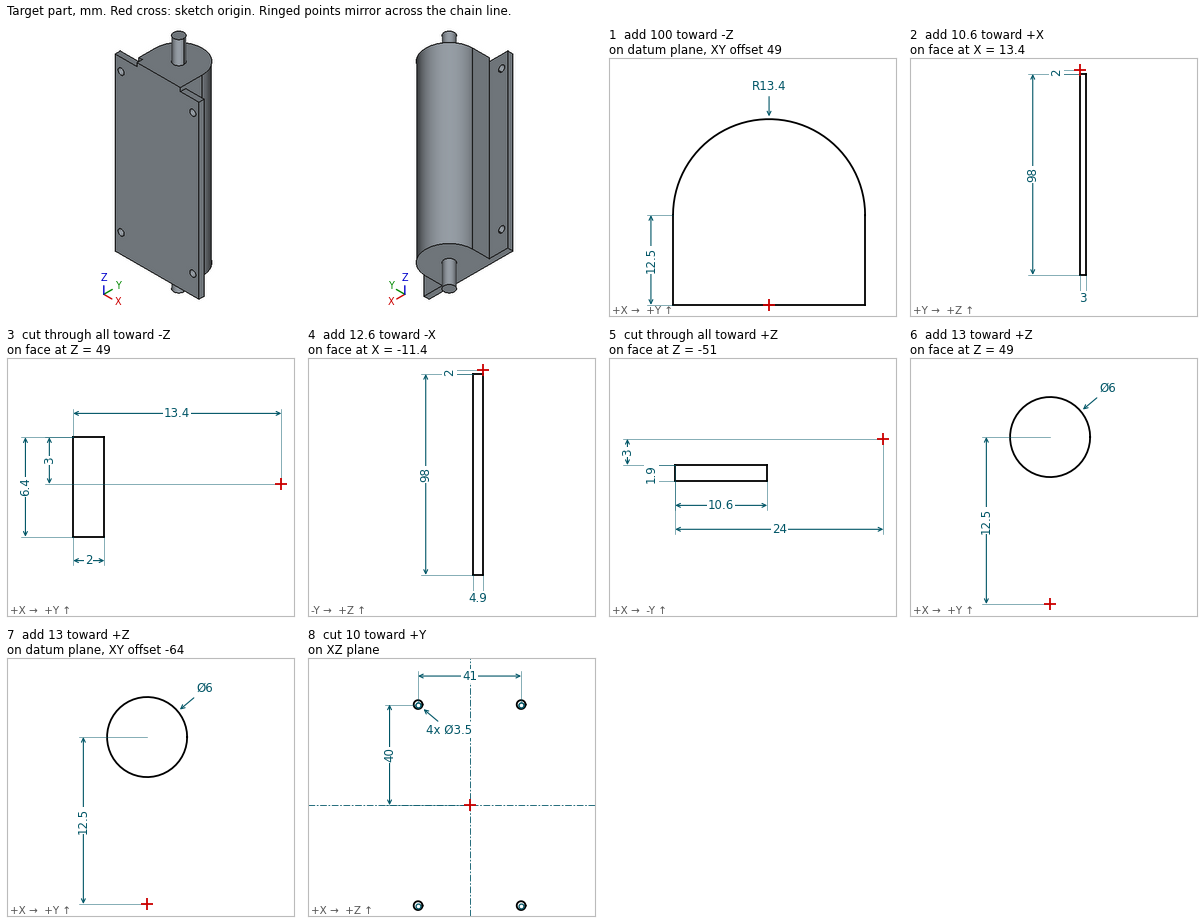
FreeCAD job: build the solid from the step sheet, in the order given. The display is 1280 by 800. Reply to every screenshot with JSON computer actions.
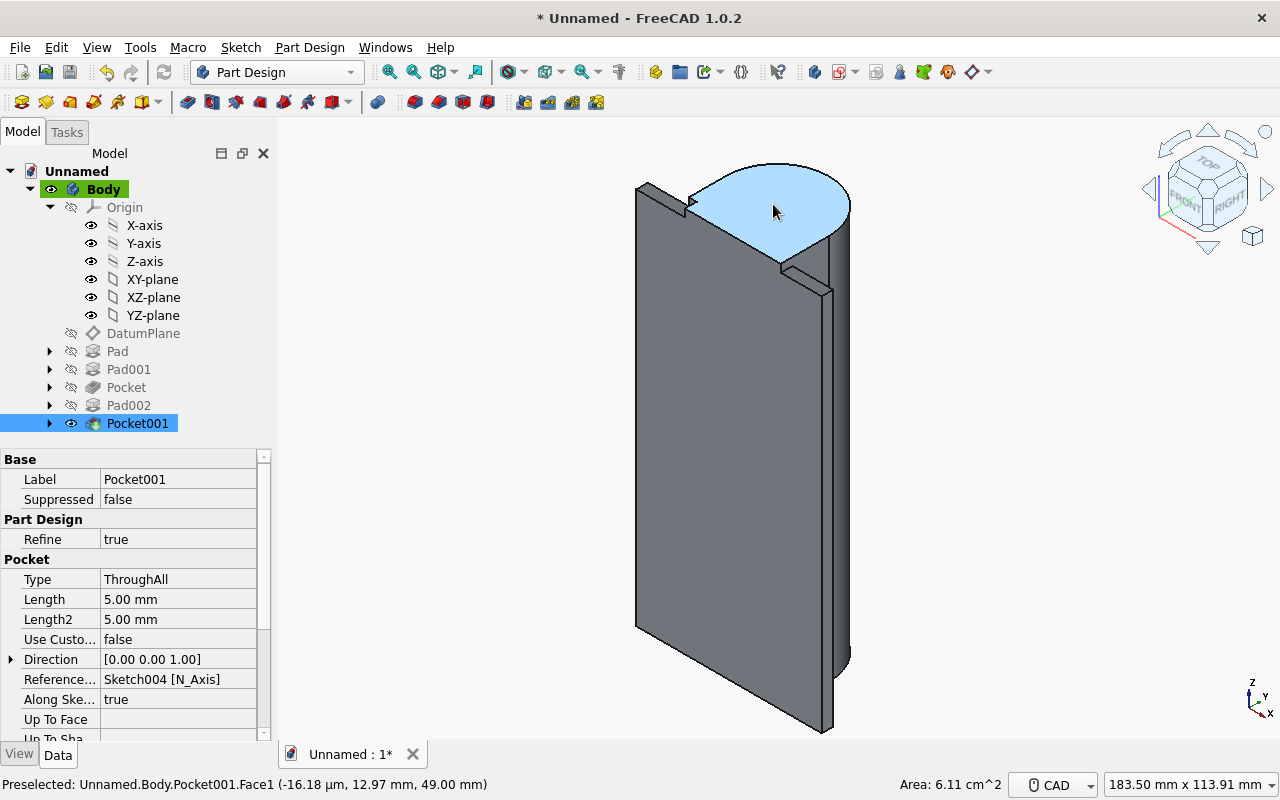
{"action": "left_click", "coordinate": [840, 72]}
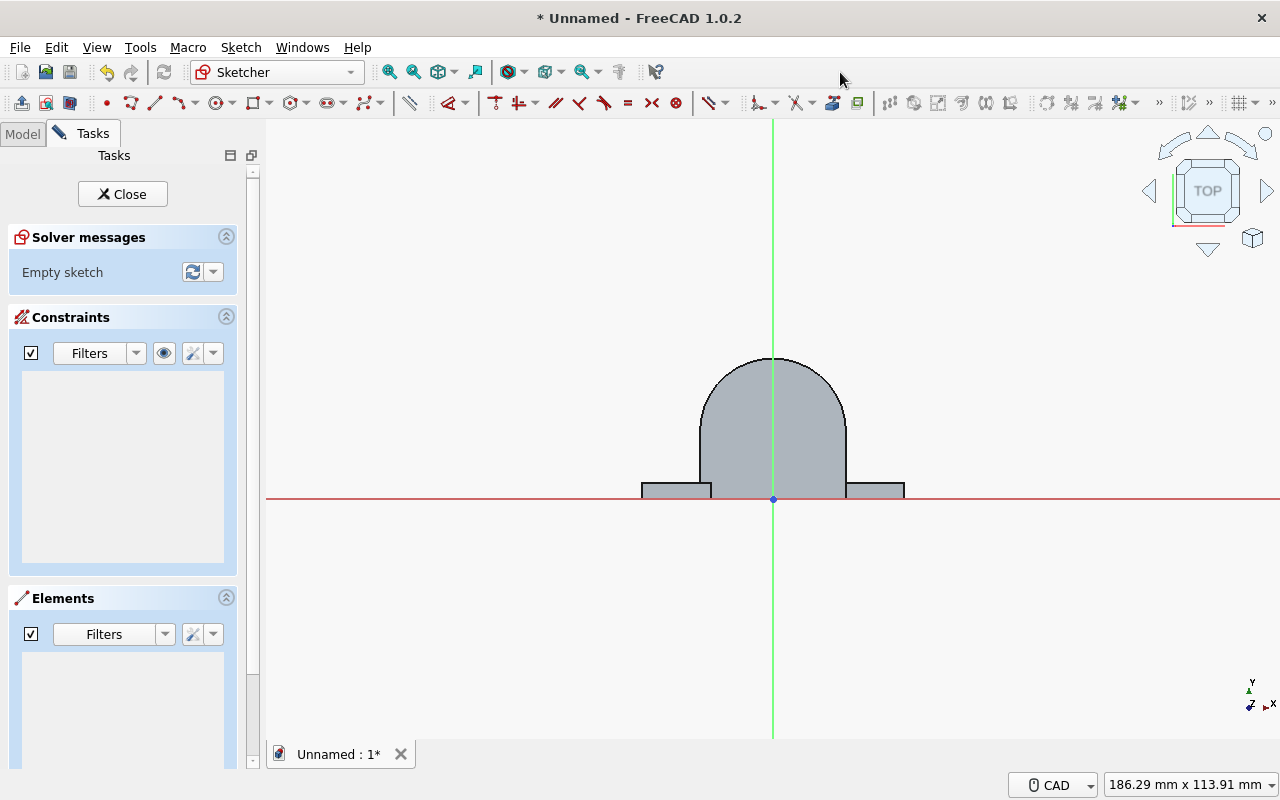
{"action": "scroll", "coordinate": [778, 432], "scroll_direction": "up", "scroll_amount": 13}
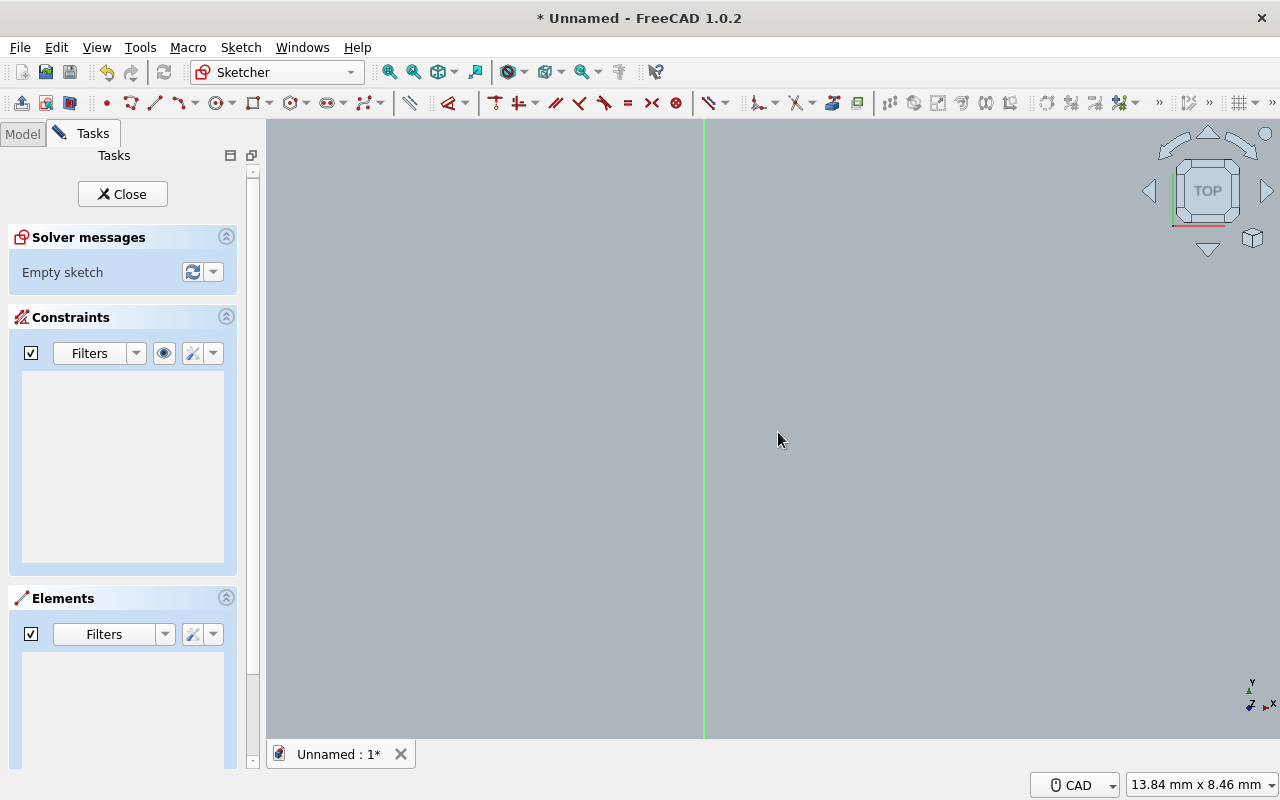
{"action": "left_click", "coordinate": [216, 104]}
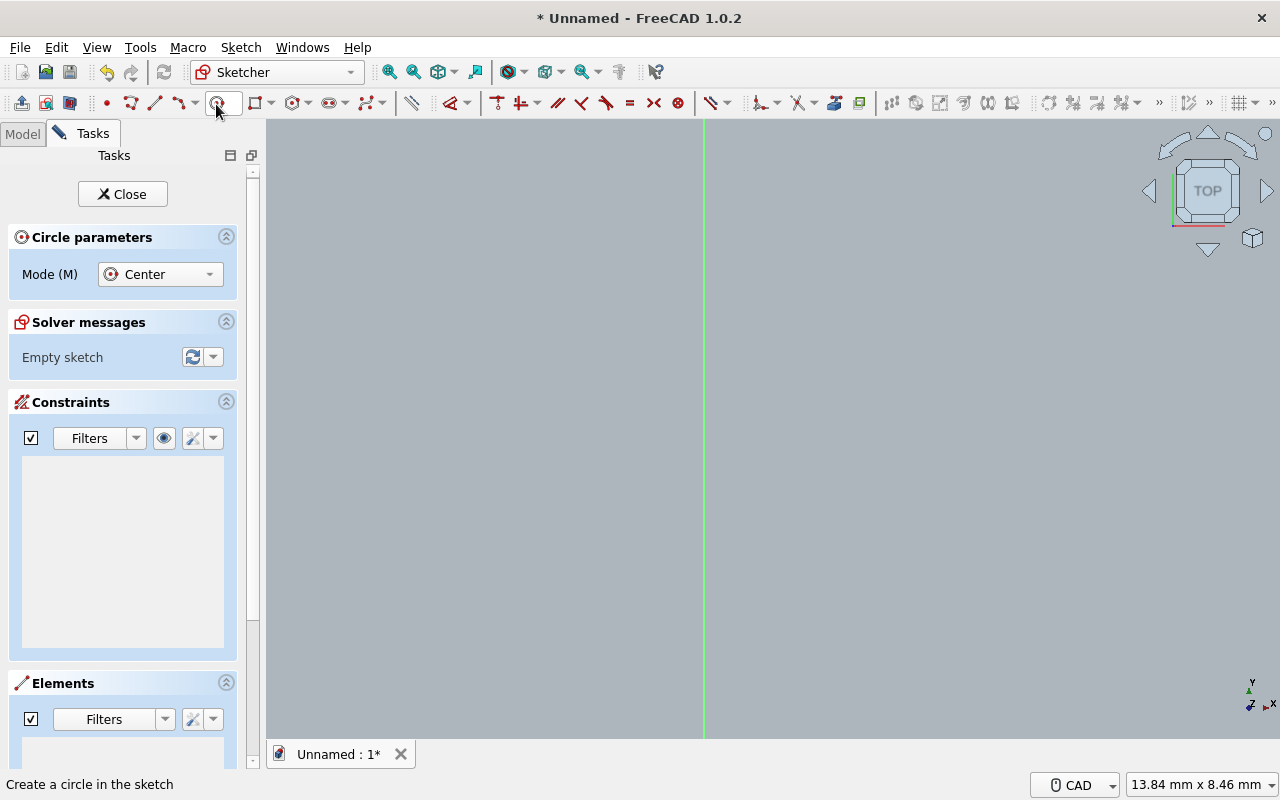
{"action": "left_click", "coordinate": [704, 418]}
{"action": "left_click", "coordinate": [860, 263]}
{"action": "key", "text": "Escape"}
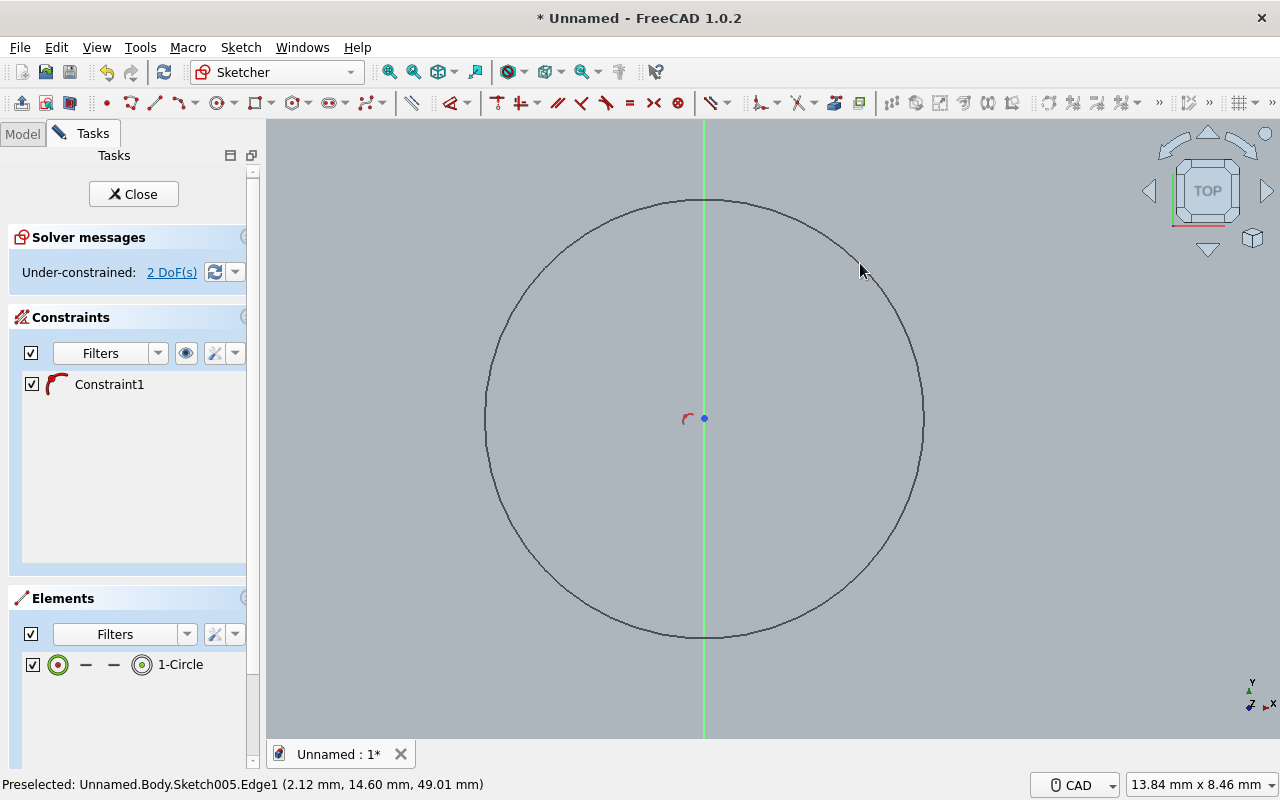
{"action": "left_click", "coordinate": [450, 104]}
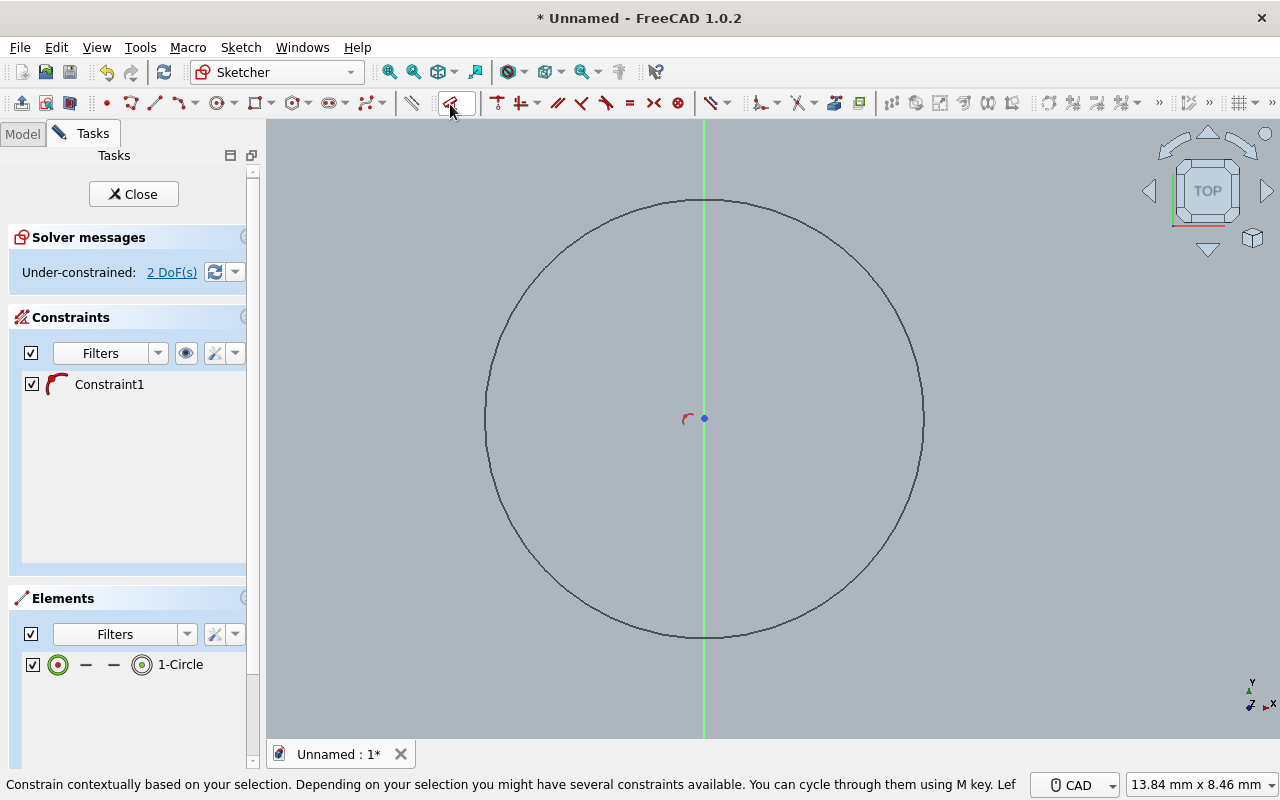
{"action": "left_click", "coordinate": [859, 263]}
{"action": "left_click", "coordinate": [882, 240]}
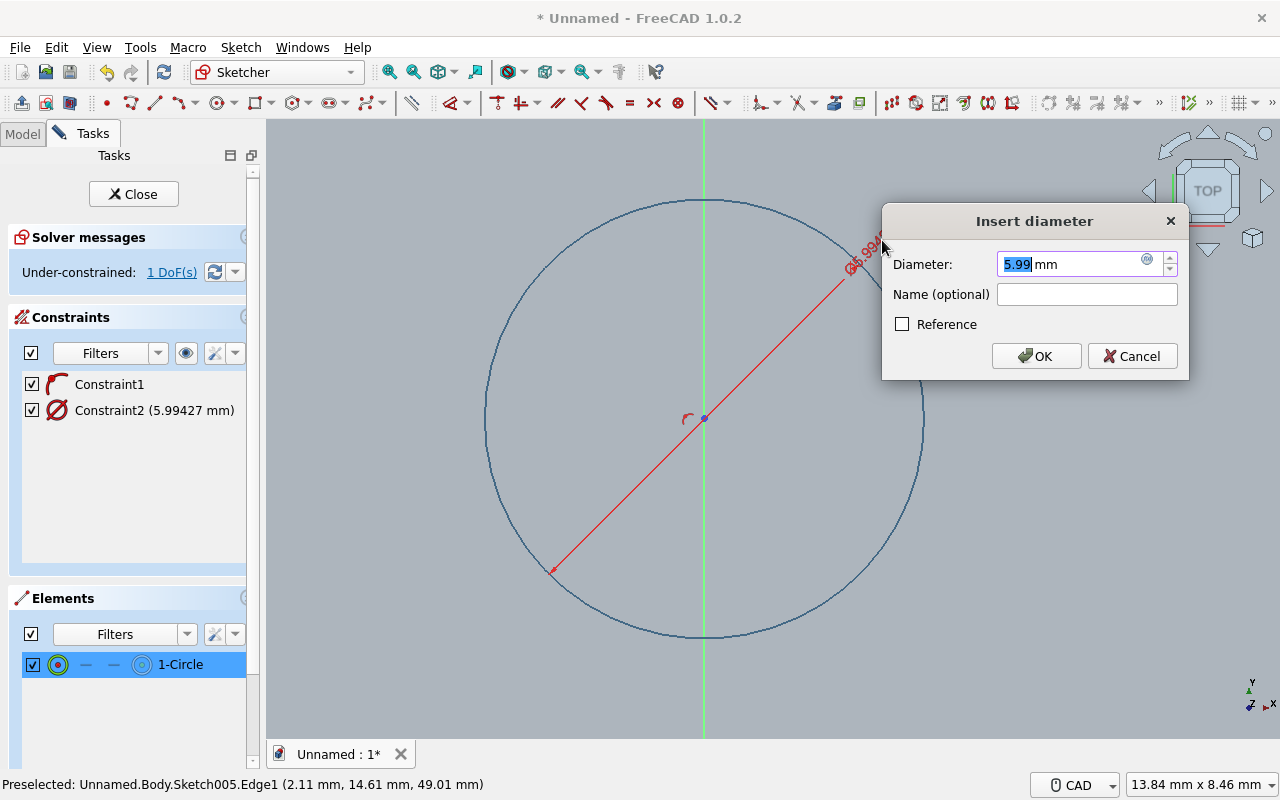
{"action": "type", "text": "6"}
{"action": "key", "text": "Return"}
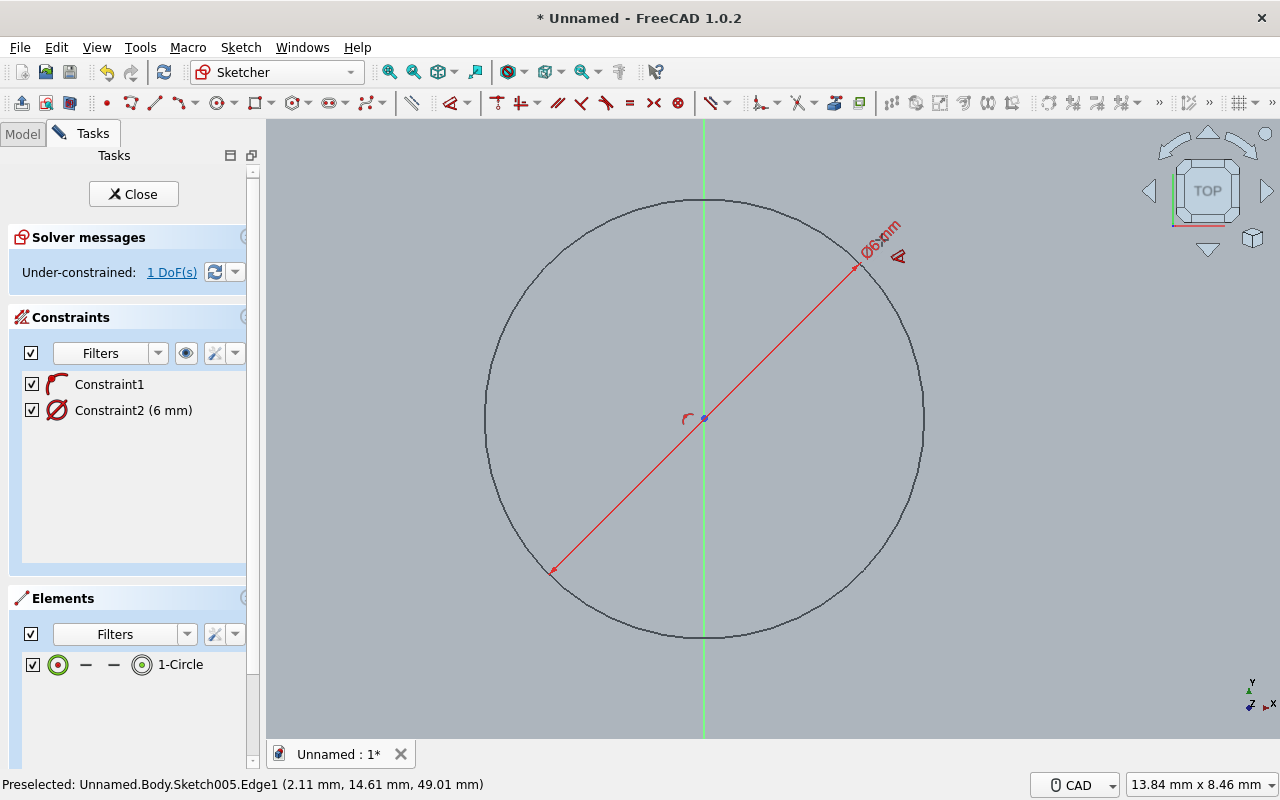
{"action": "left_click", "coordinate": [704, 419]}
{"action": "left_click", "coordinate": [738, 565]}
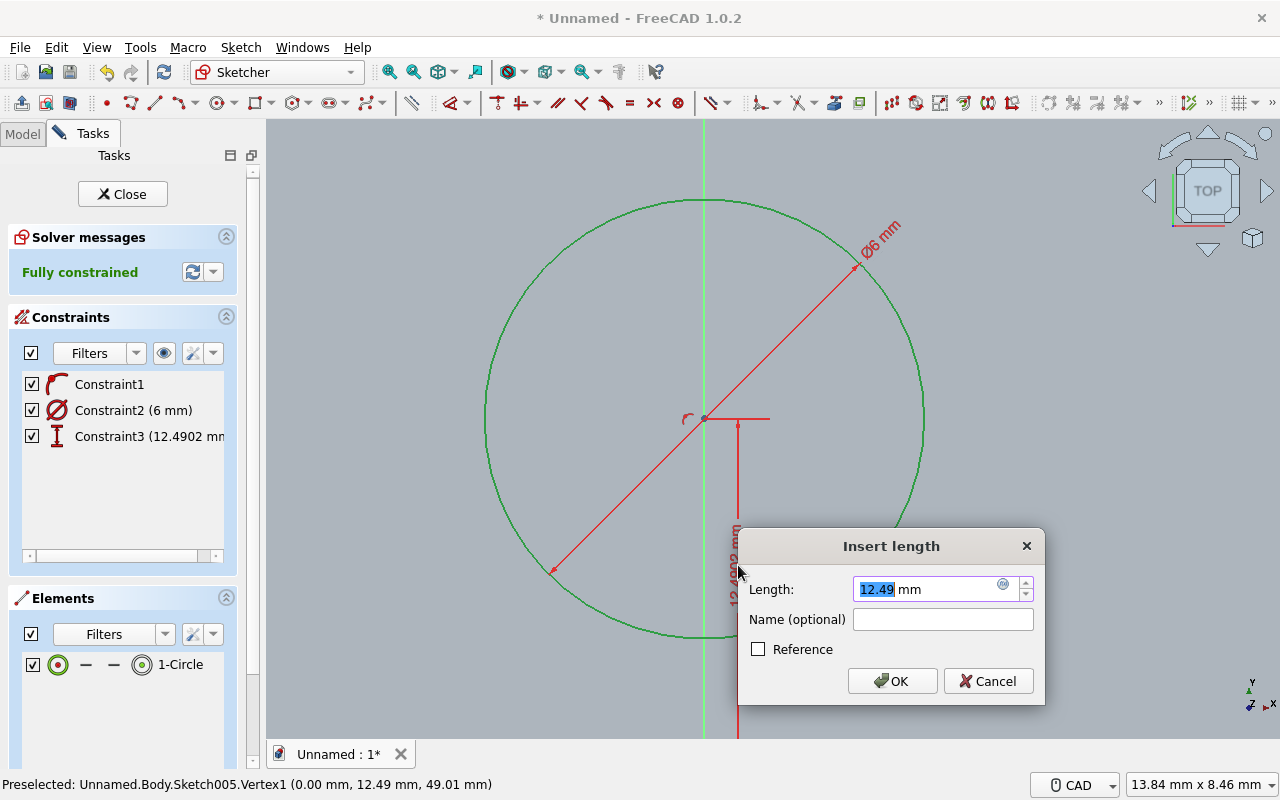
{"action": "type", "text": "12.5"}
{"action": "key", "text": "Return"}
{"action": "key", "text": "Escape"}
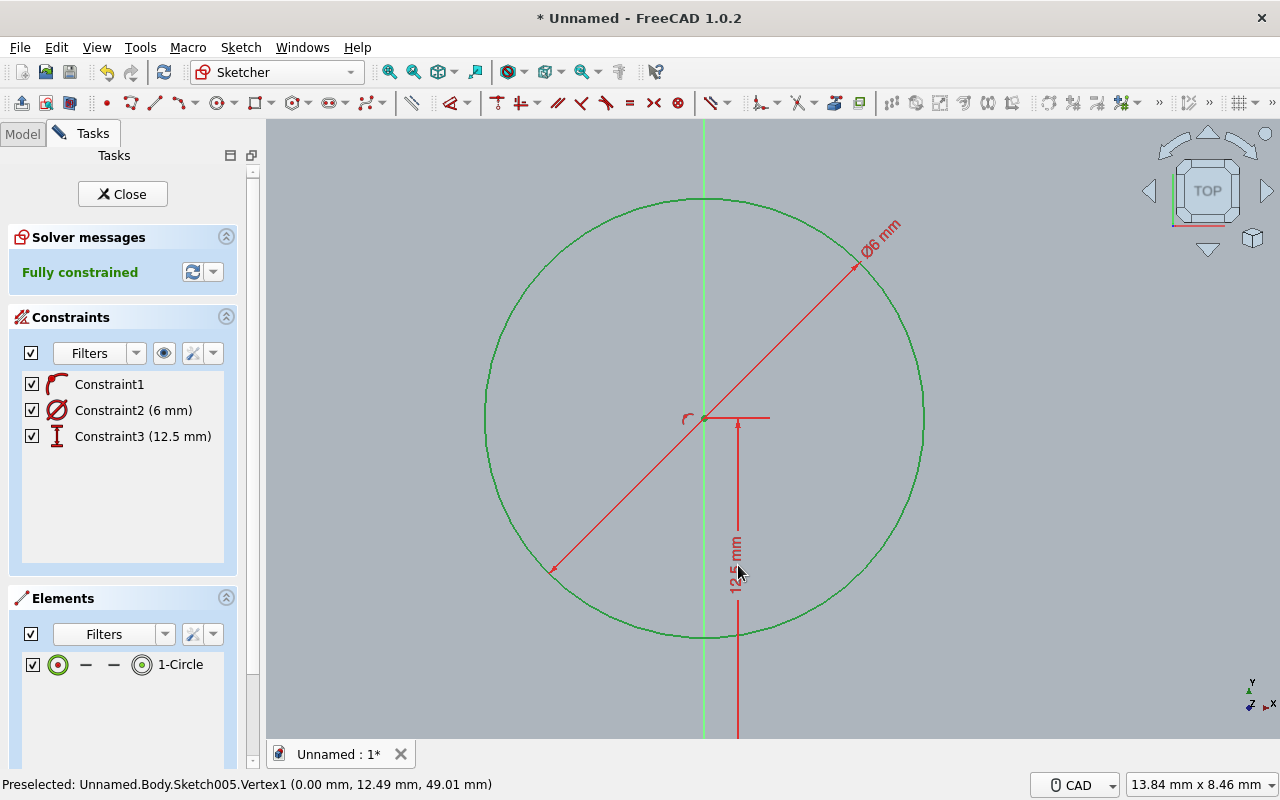
{"action": "left_click", "coordinate": [123, 194]}